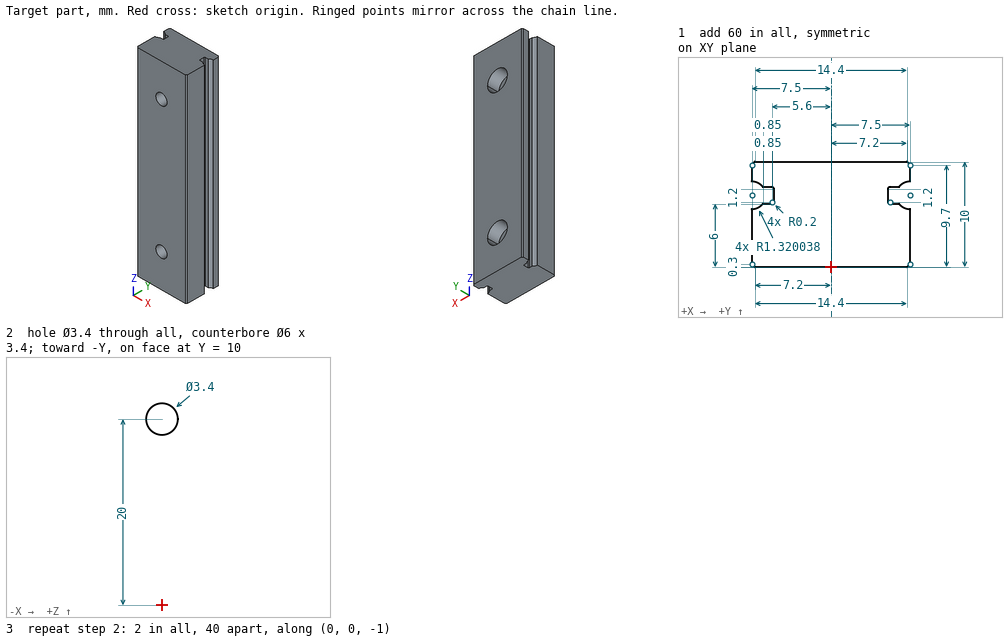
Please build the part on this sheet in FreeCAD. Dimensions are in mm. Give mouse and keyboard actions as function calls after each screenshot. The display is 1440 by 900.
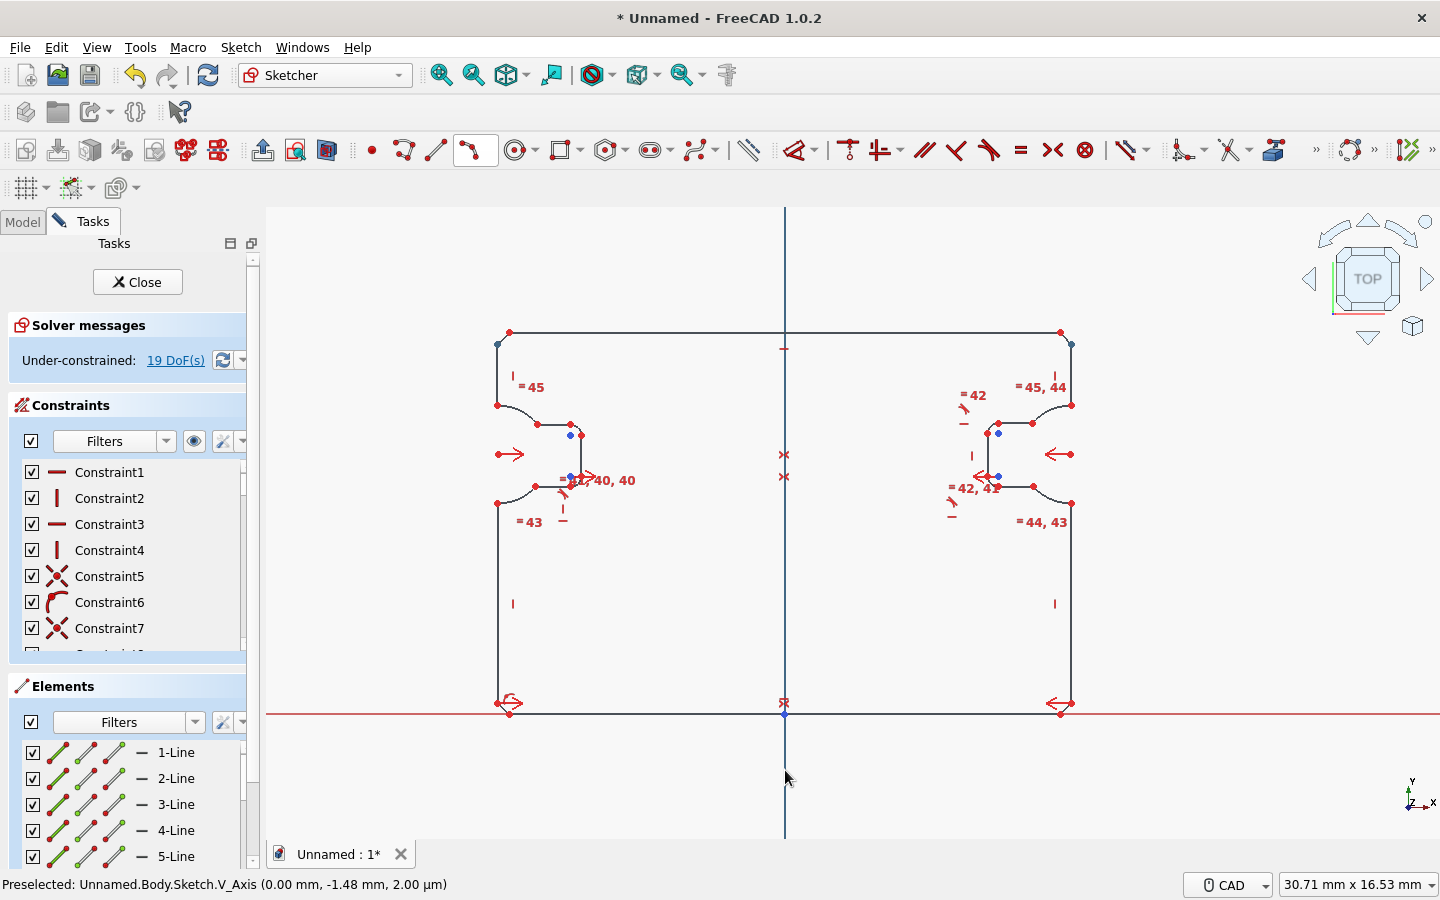
key(s)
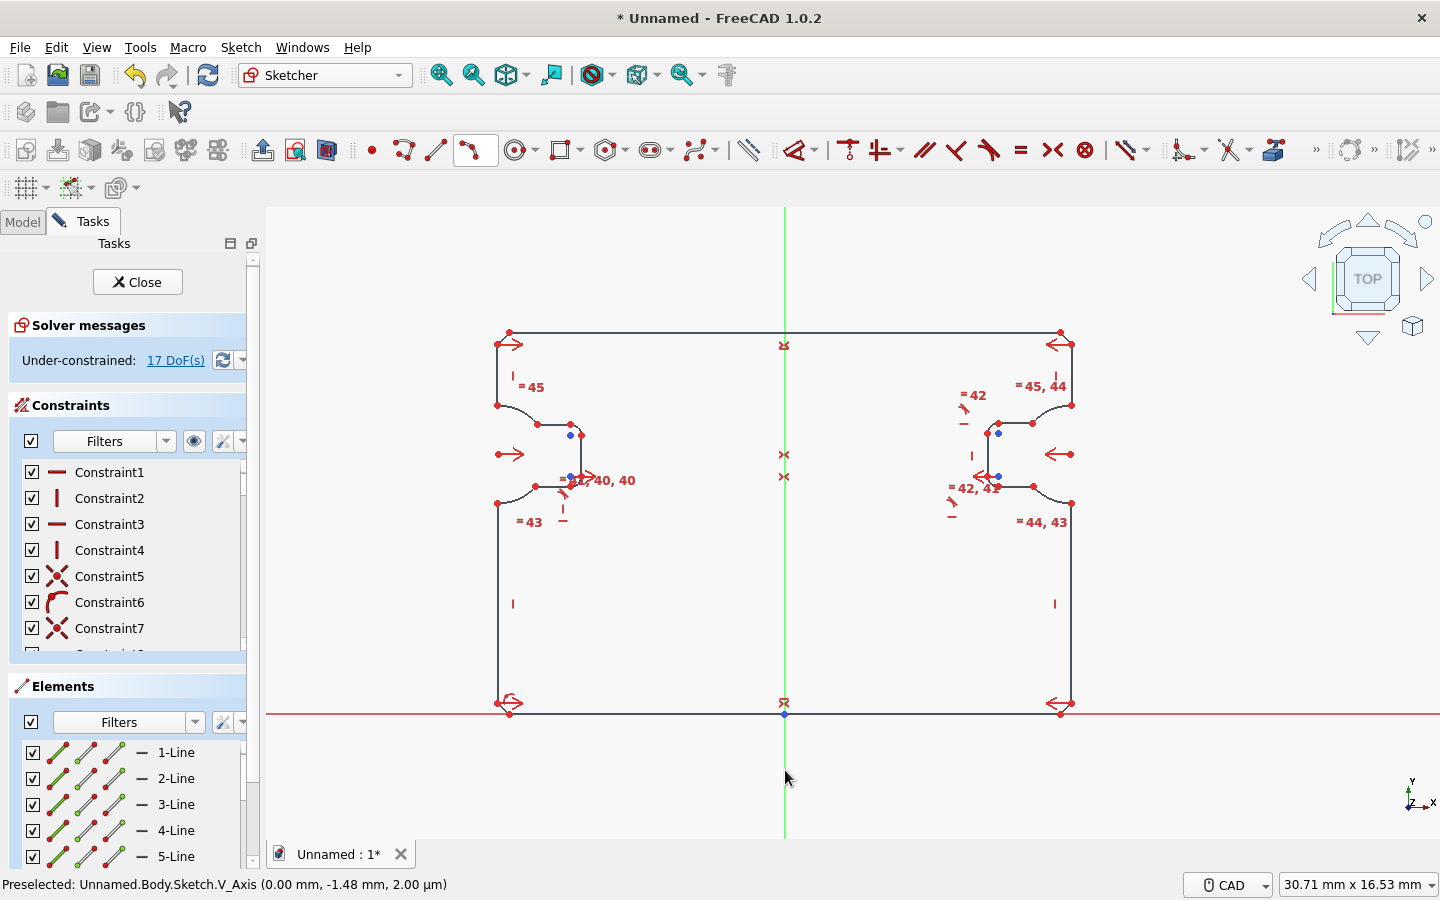
click(794, 150)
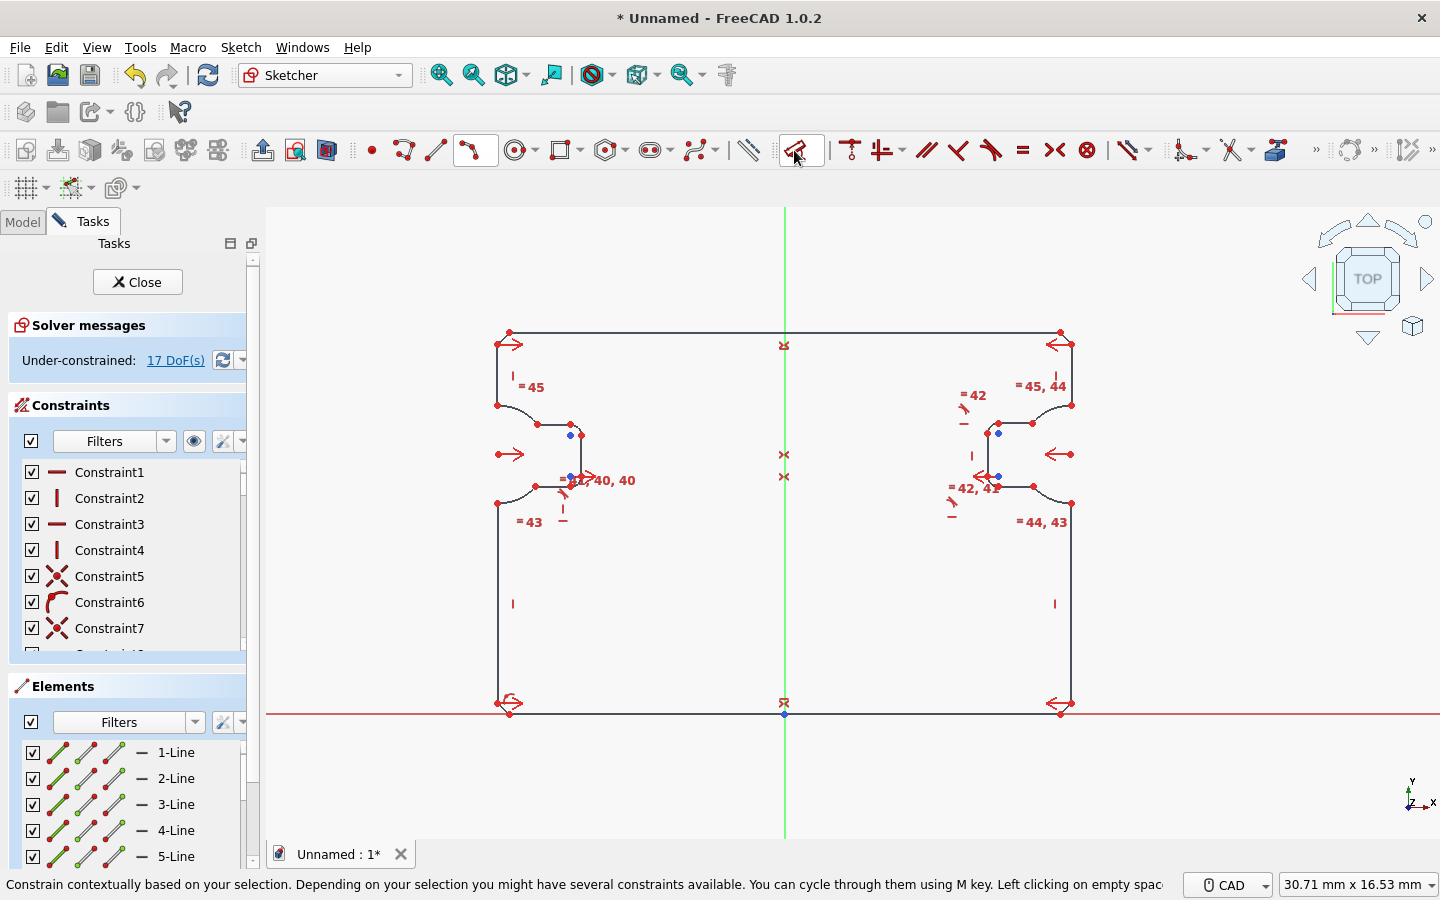
scroll(578, 428, up, 9)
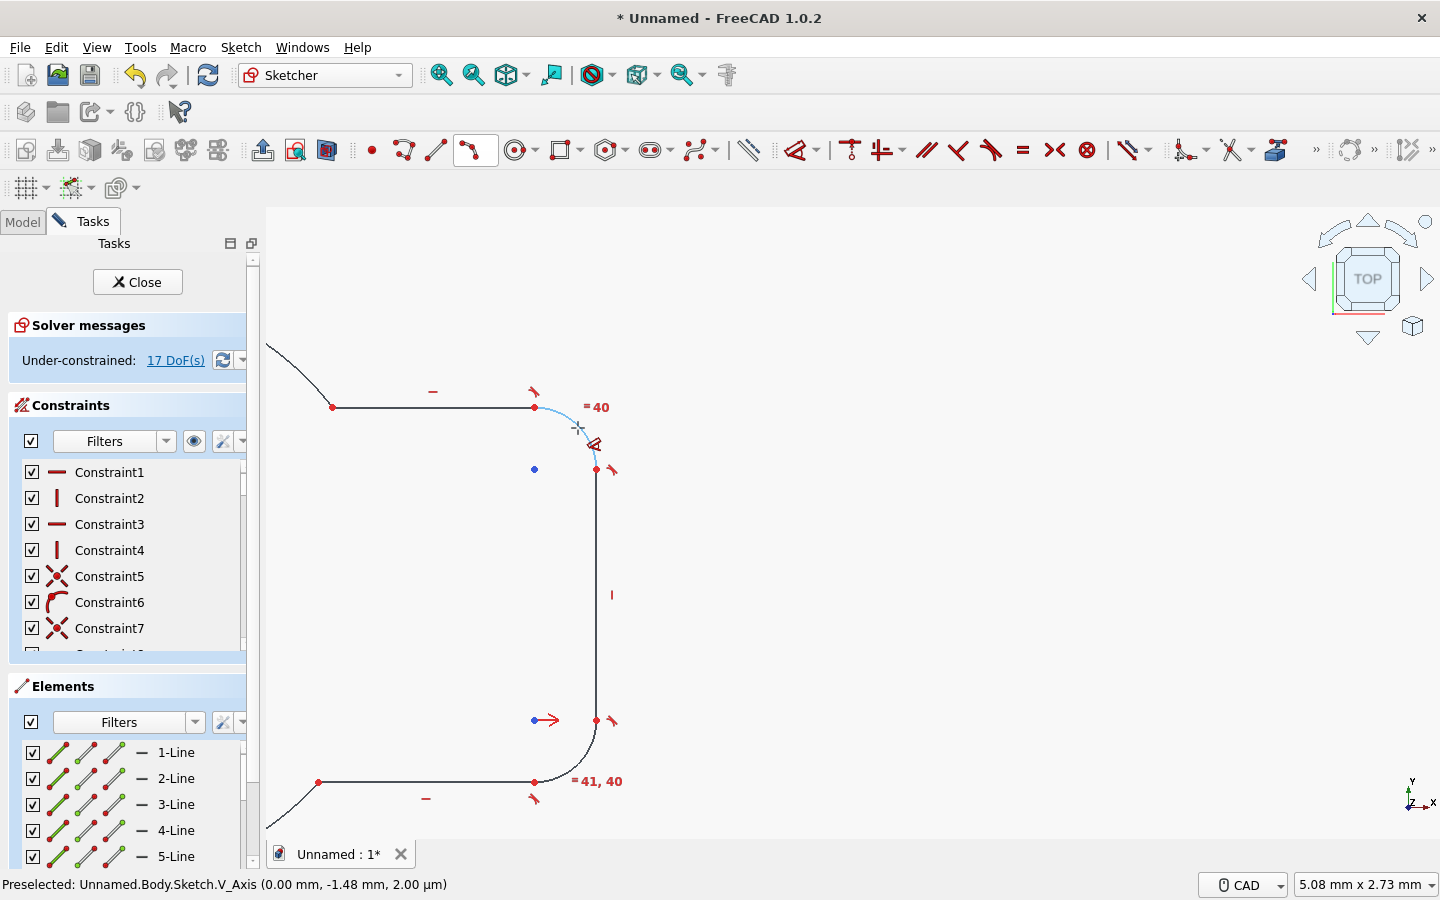
click(578, 426)
click(601, 403)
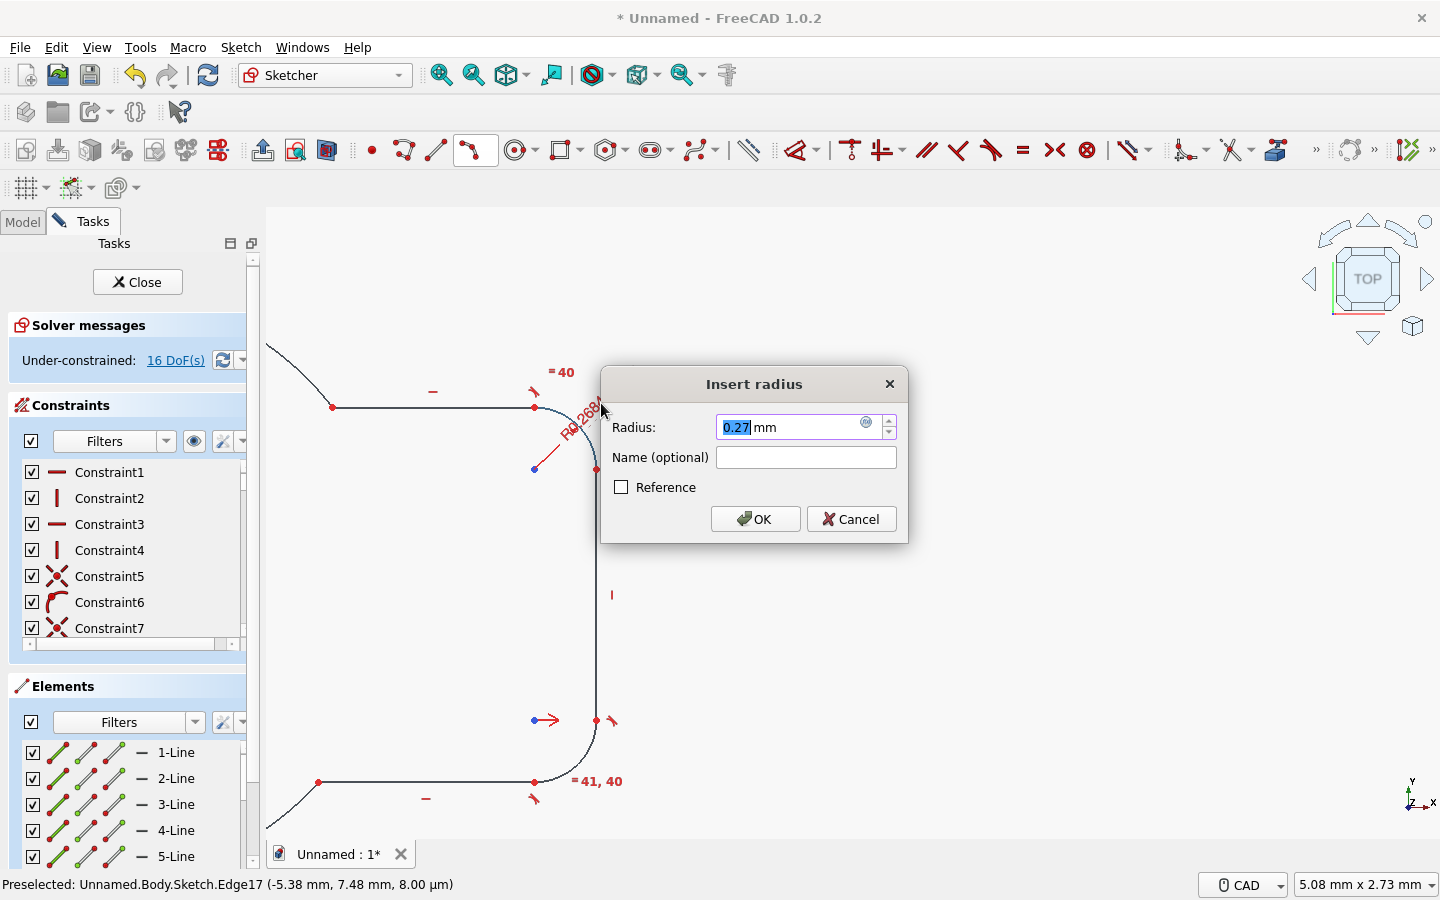
text(0.2)
key(Return)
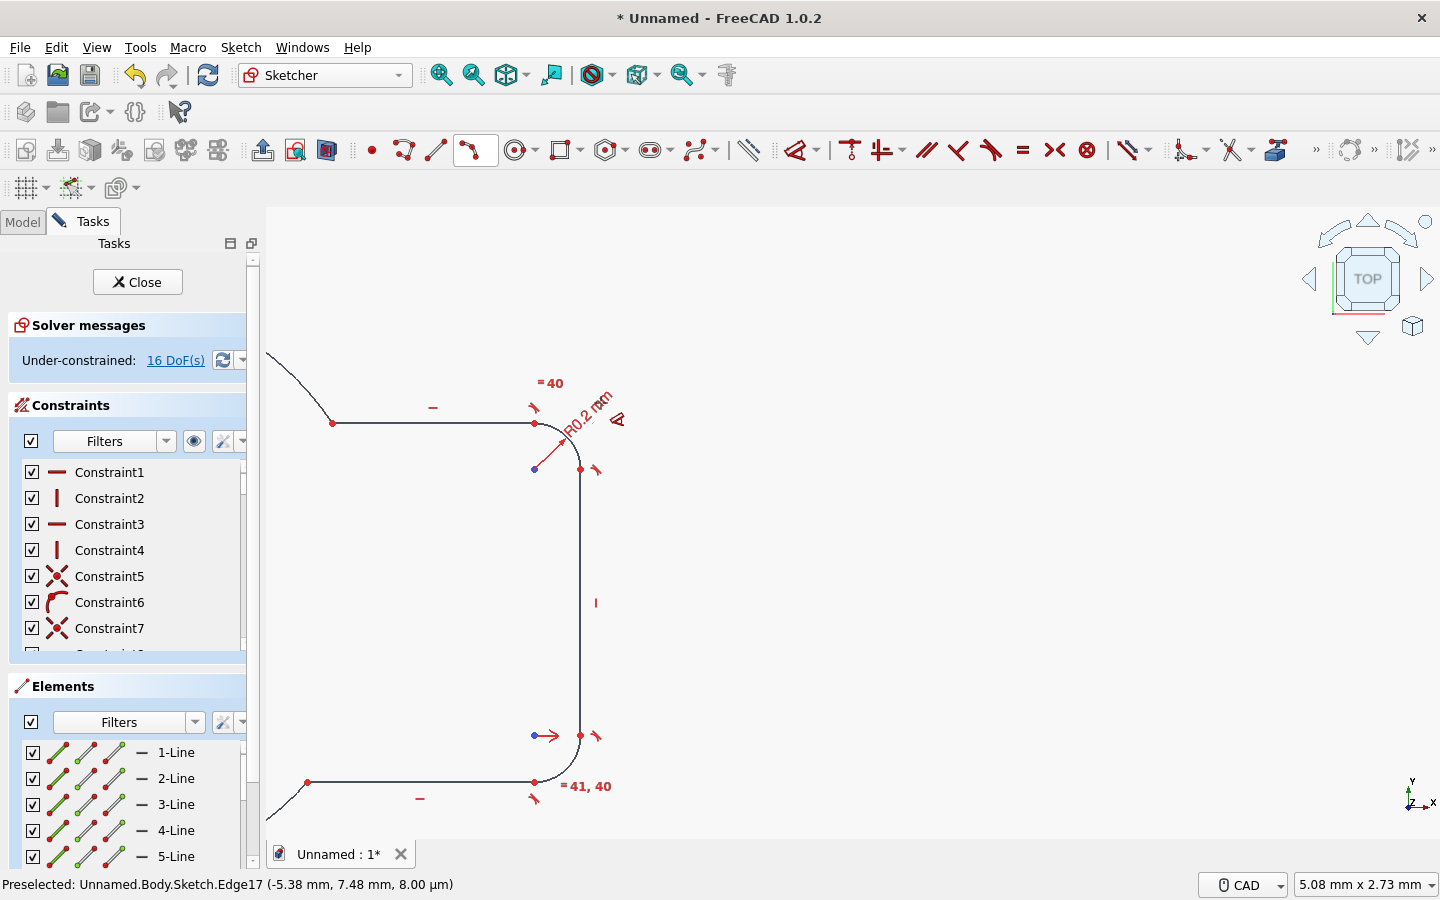
scroll(578, 428, down, 9)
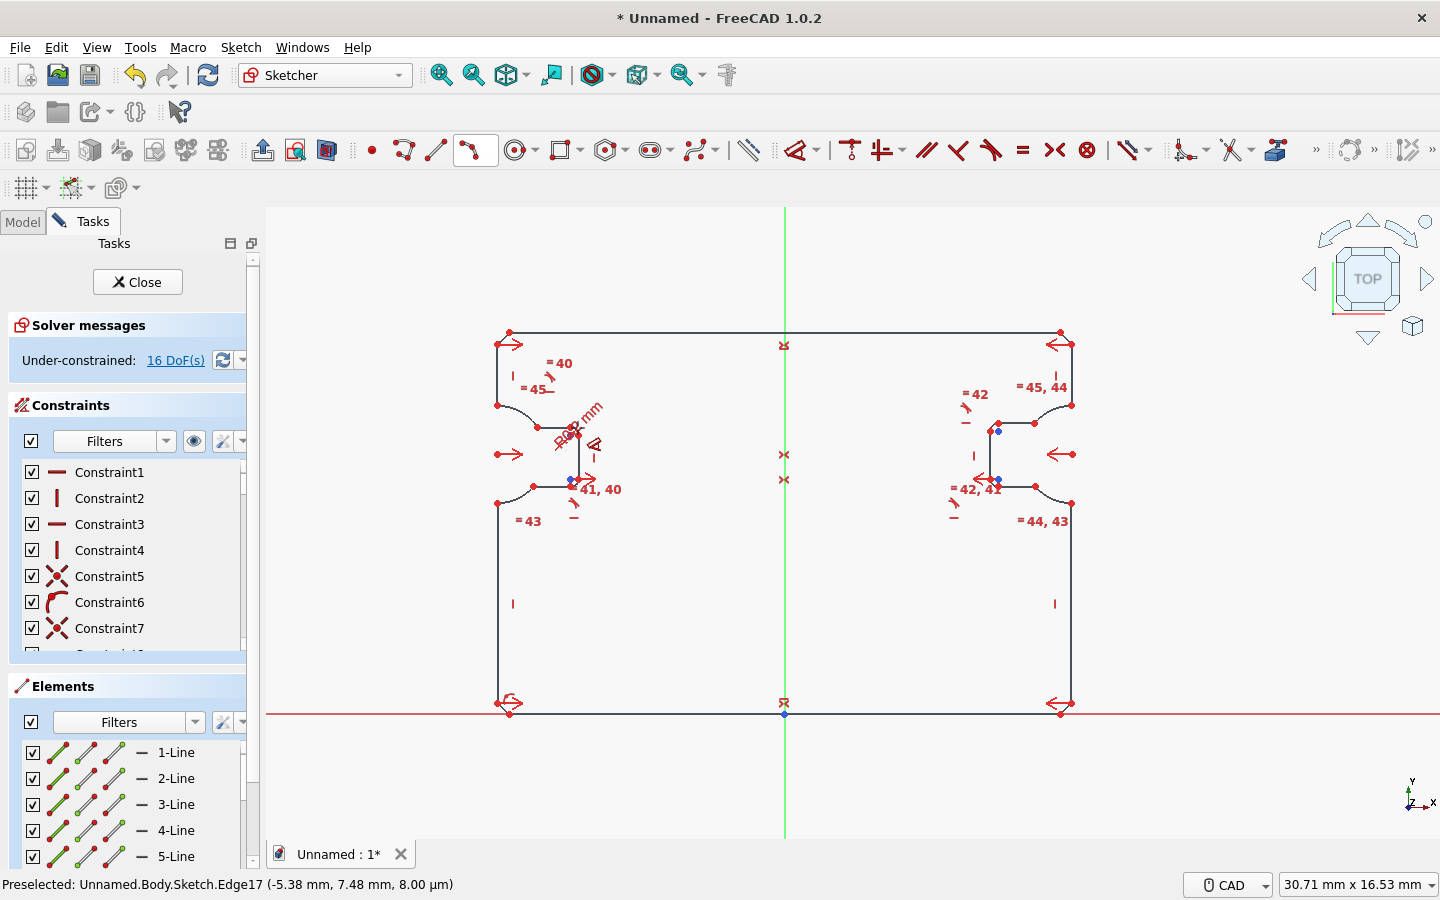
click(510, 502)
click(518, 533)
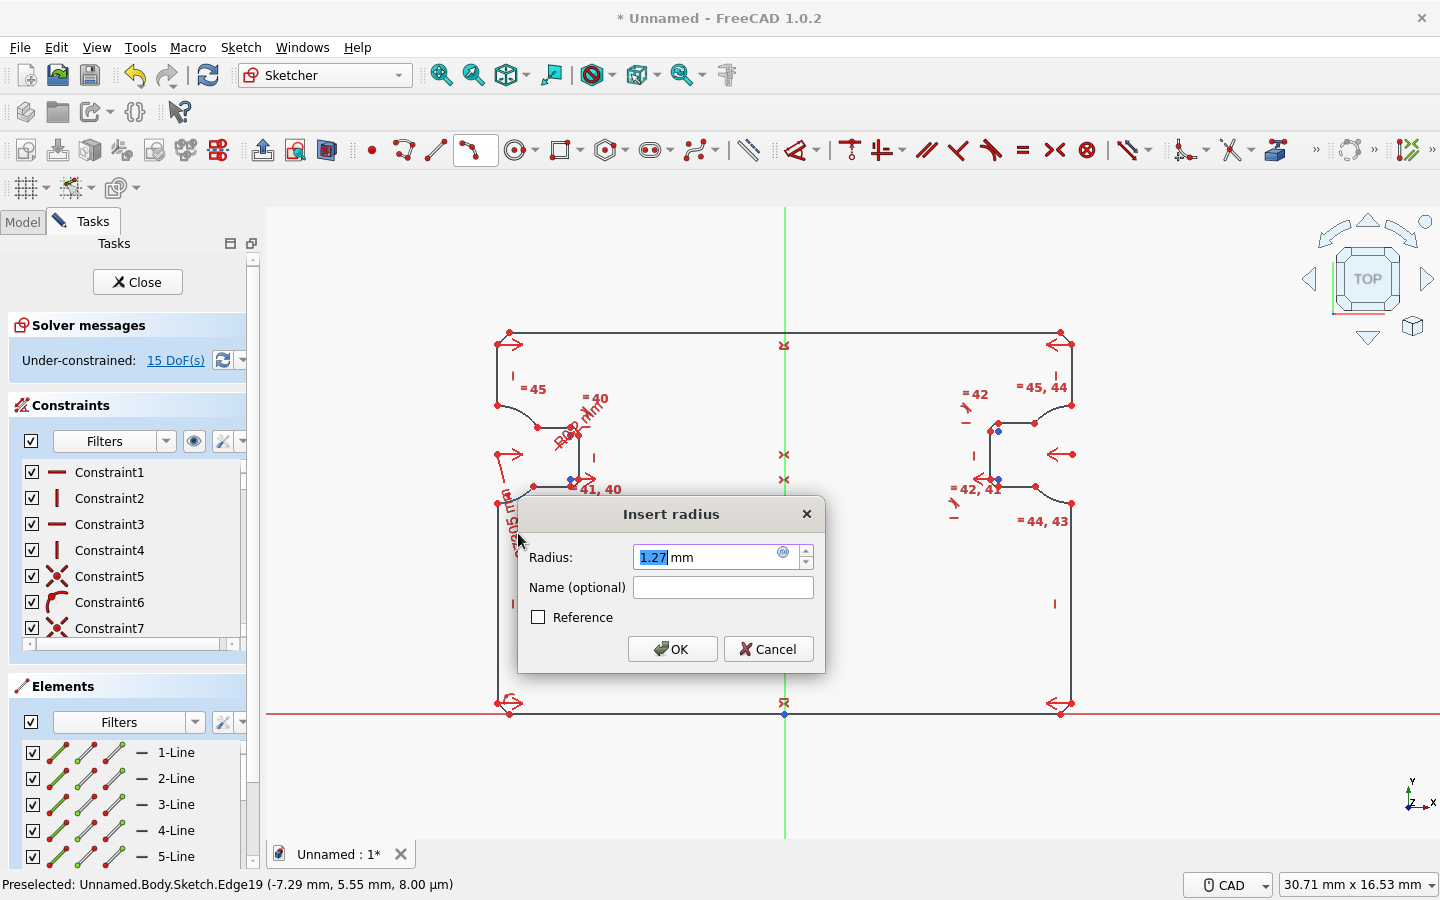
text(1.320038)
key(Return)